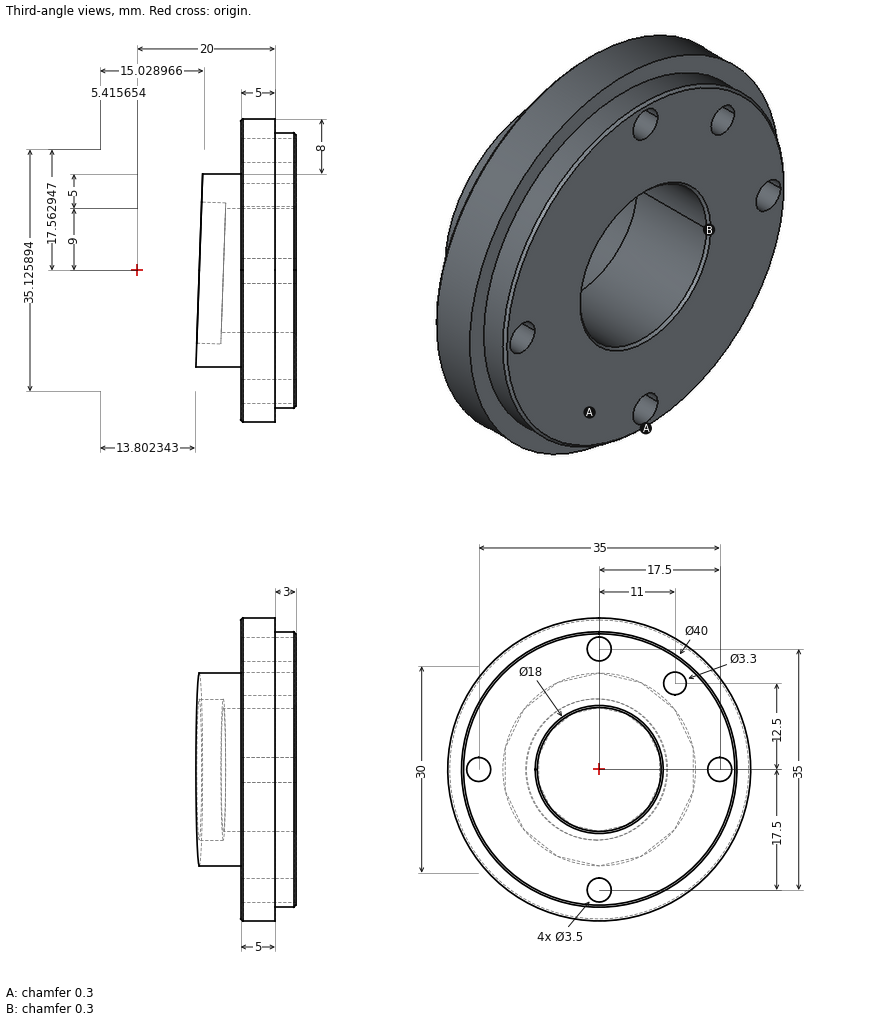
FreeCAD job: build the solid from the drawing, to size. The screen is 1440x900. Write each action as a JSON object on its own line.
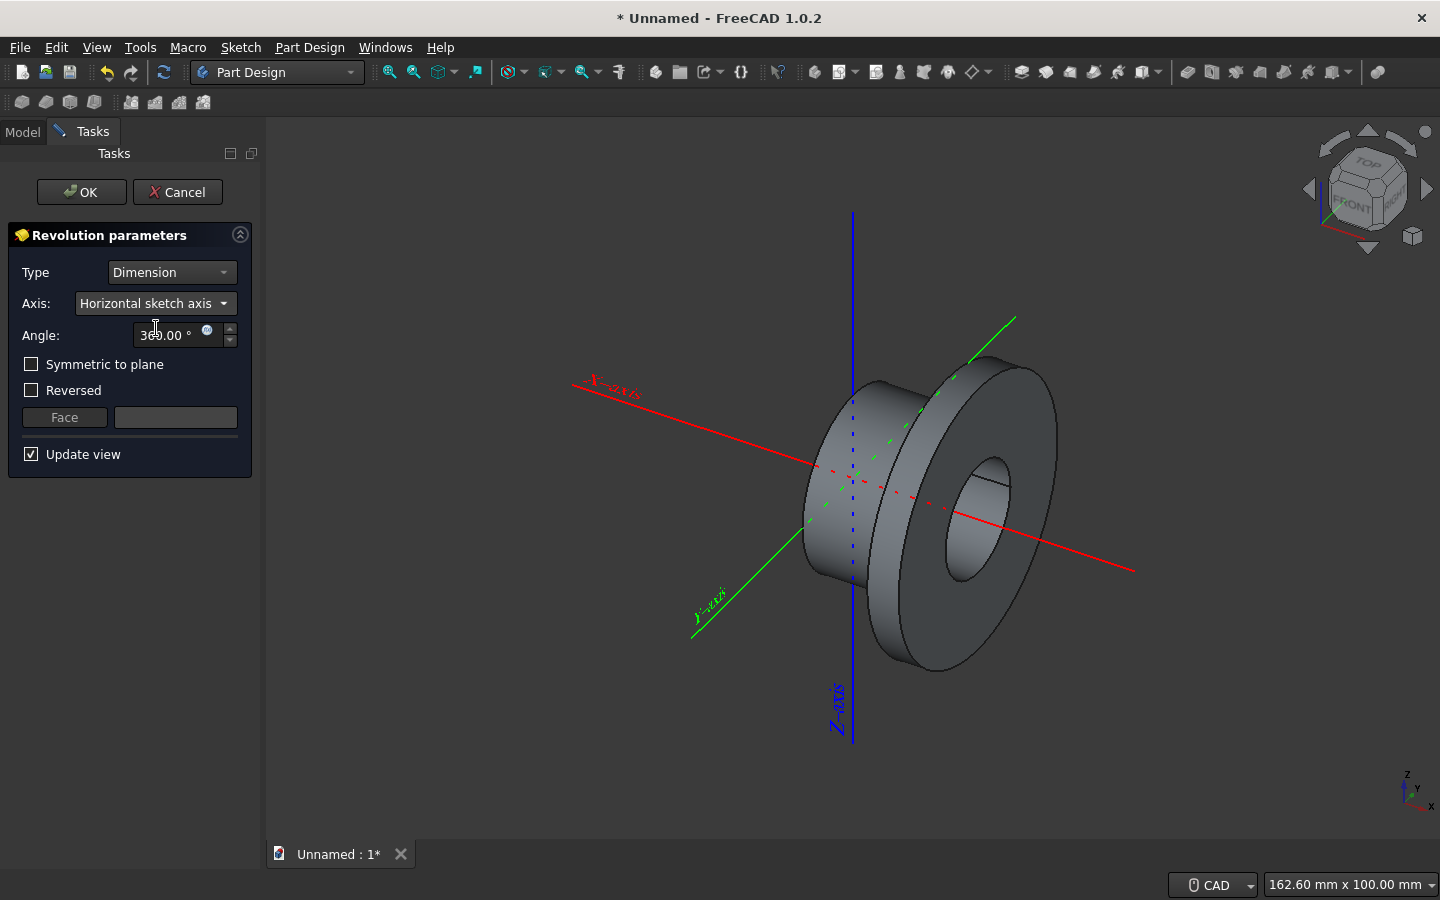
{"action": "left_click", "coordinate": [82, 192]}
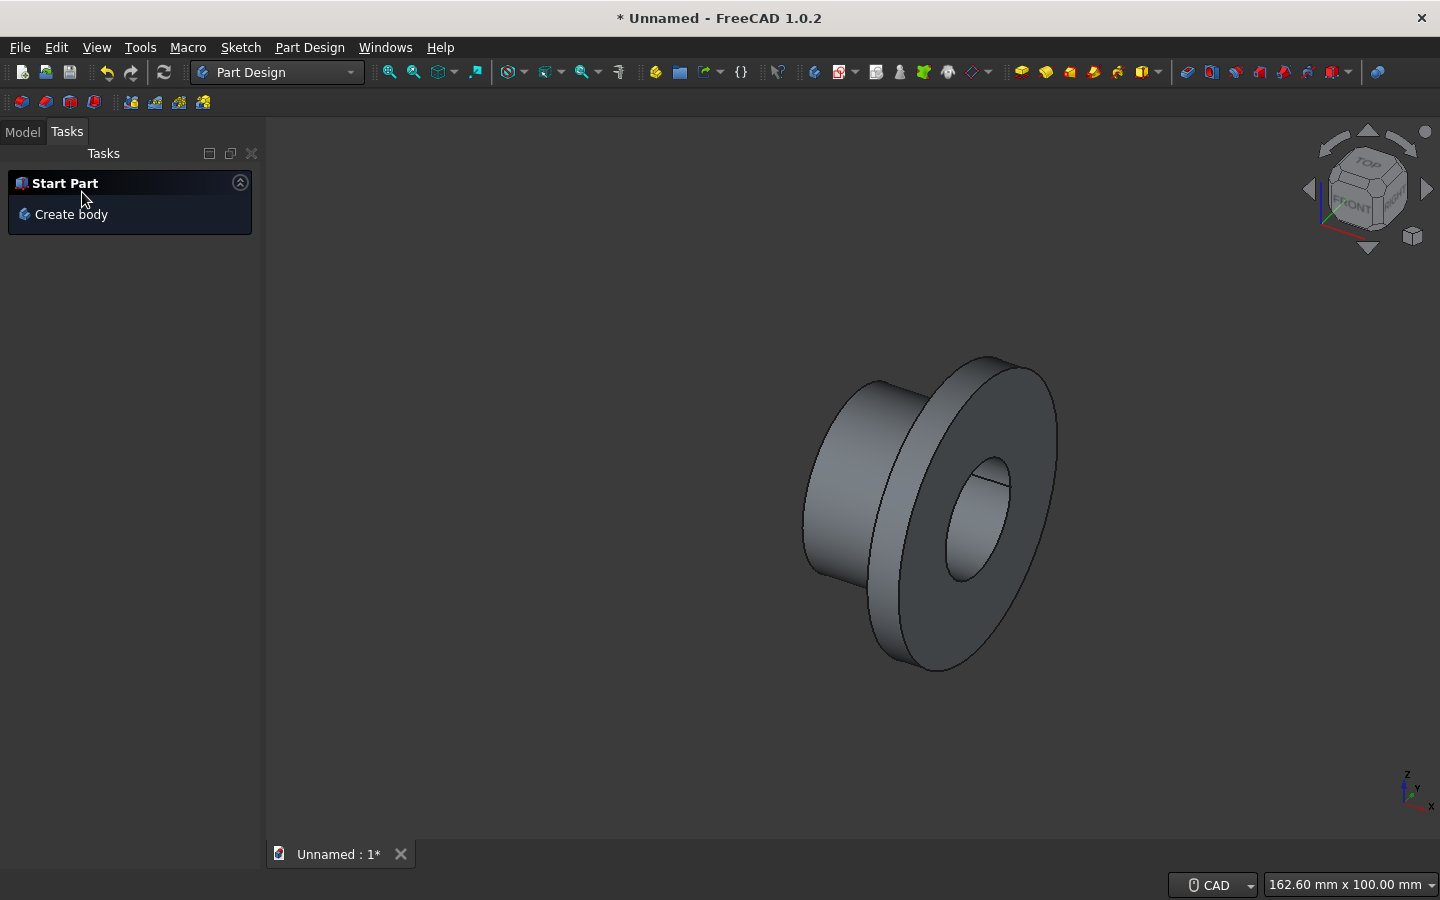
{"action": "left_click", "coordinate": [840, 72]}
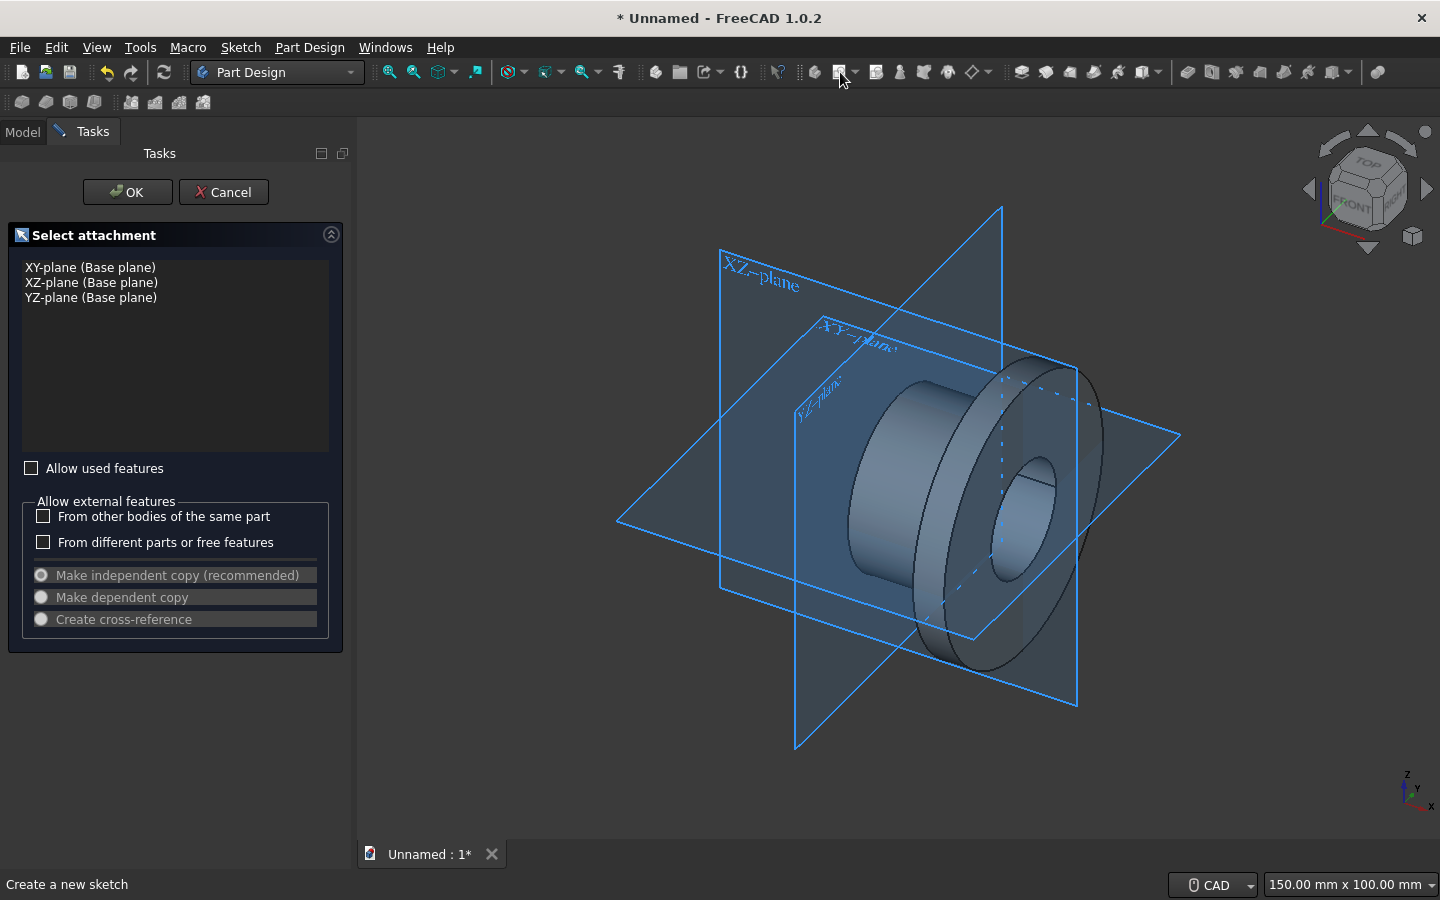
{"action": "left_click", "coordinate": [82, 268]}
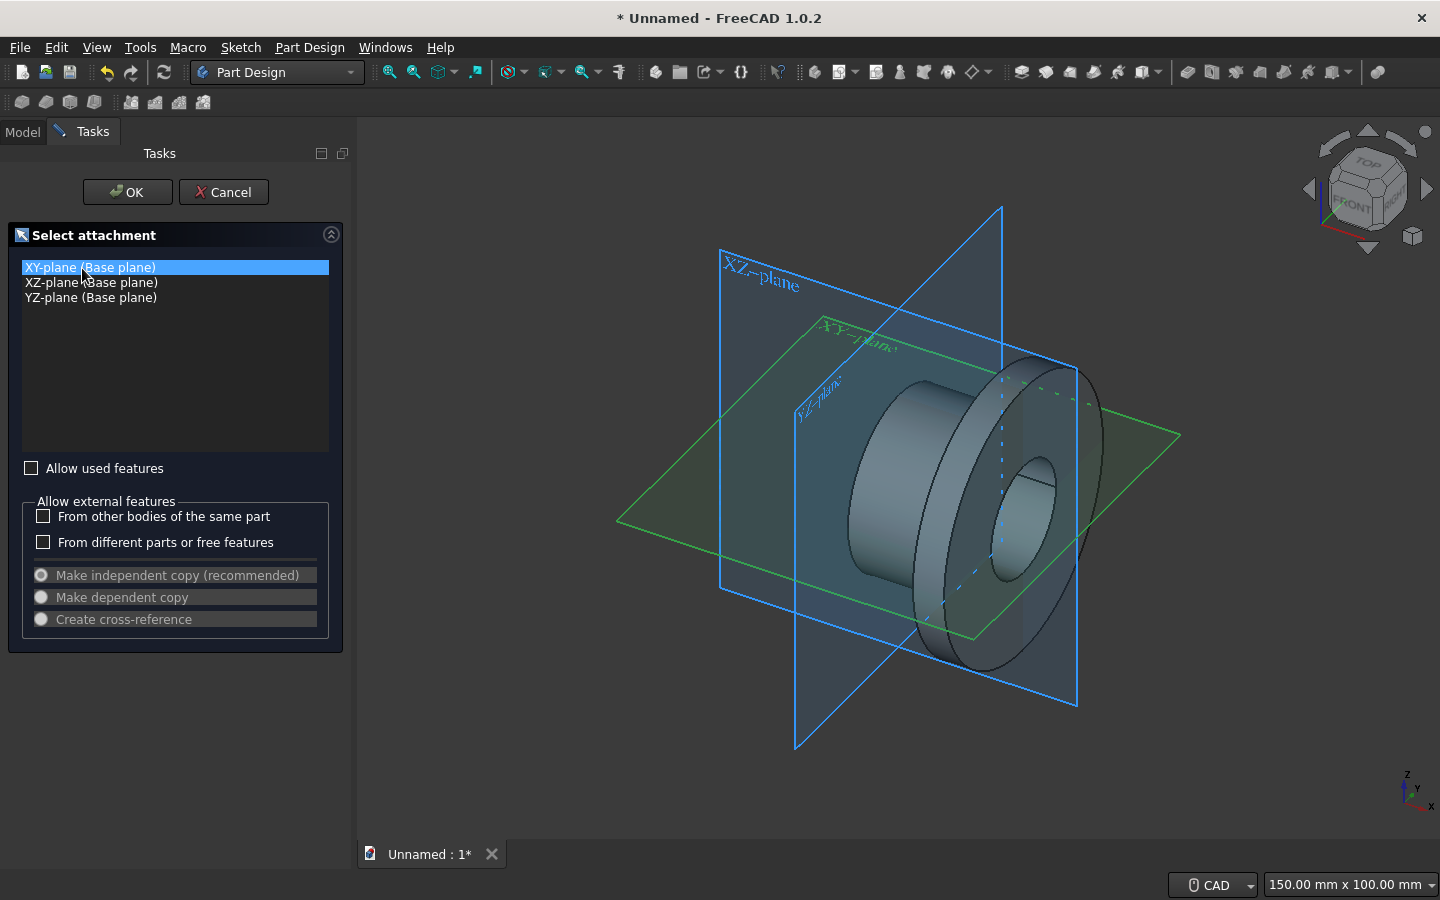
{"action": "left_click", "coordinate": [128, 192]}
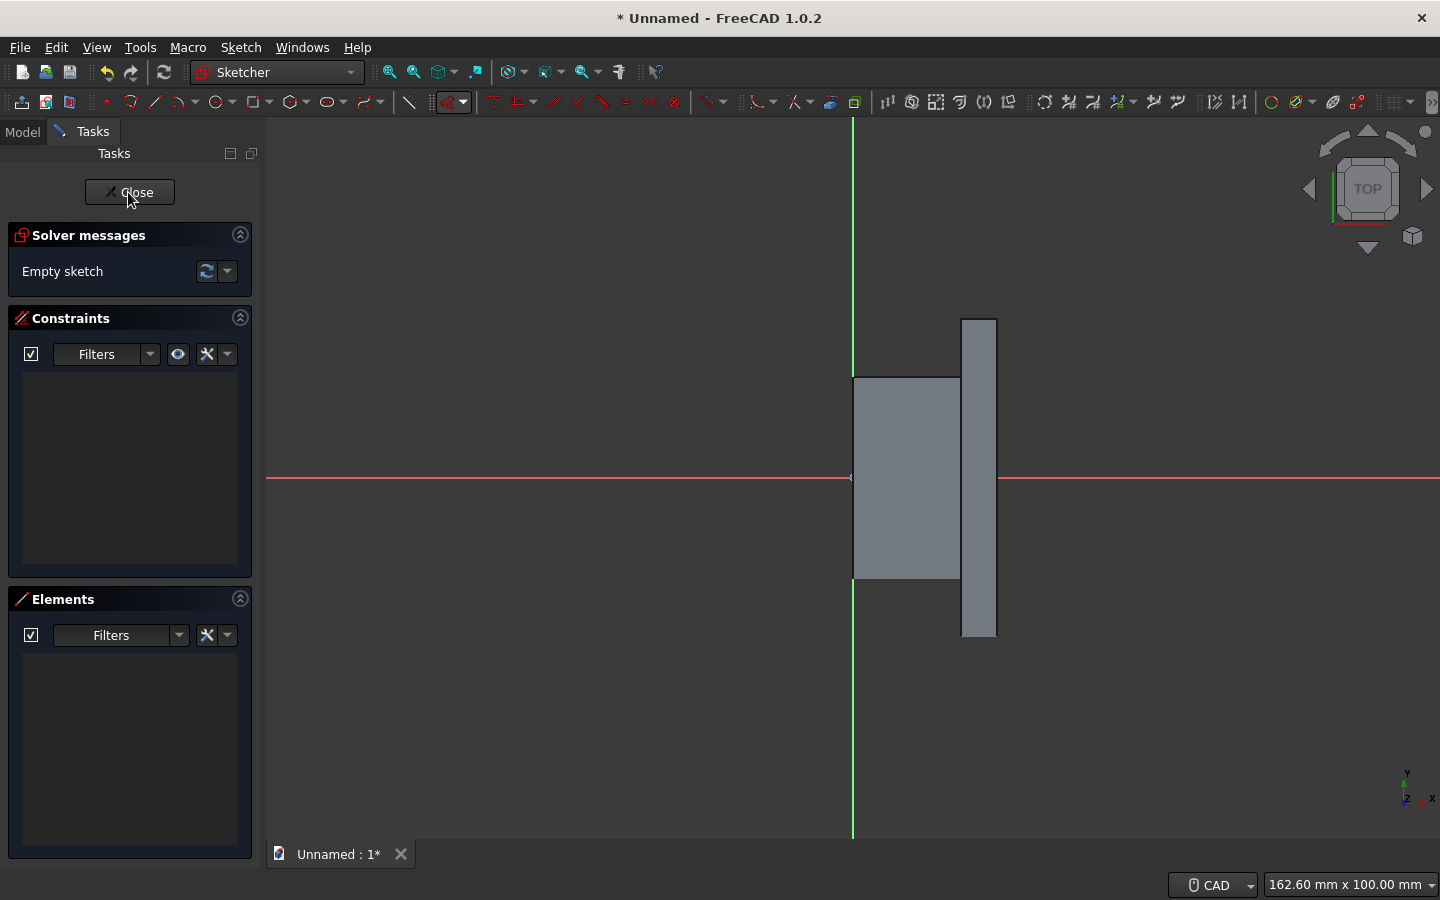
{"action": "key", "text": "q s"}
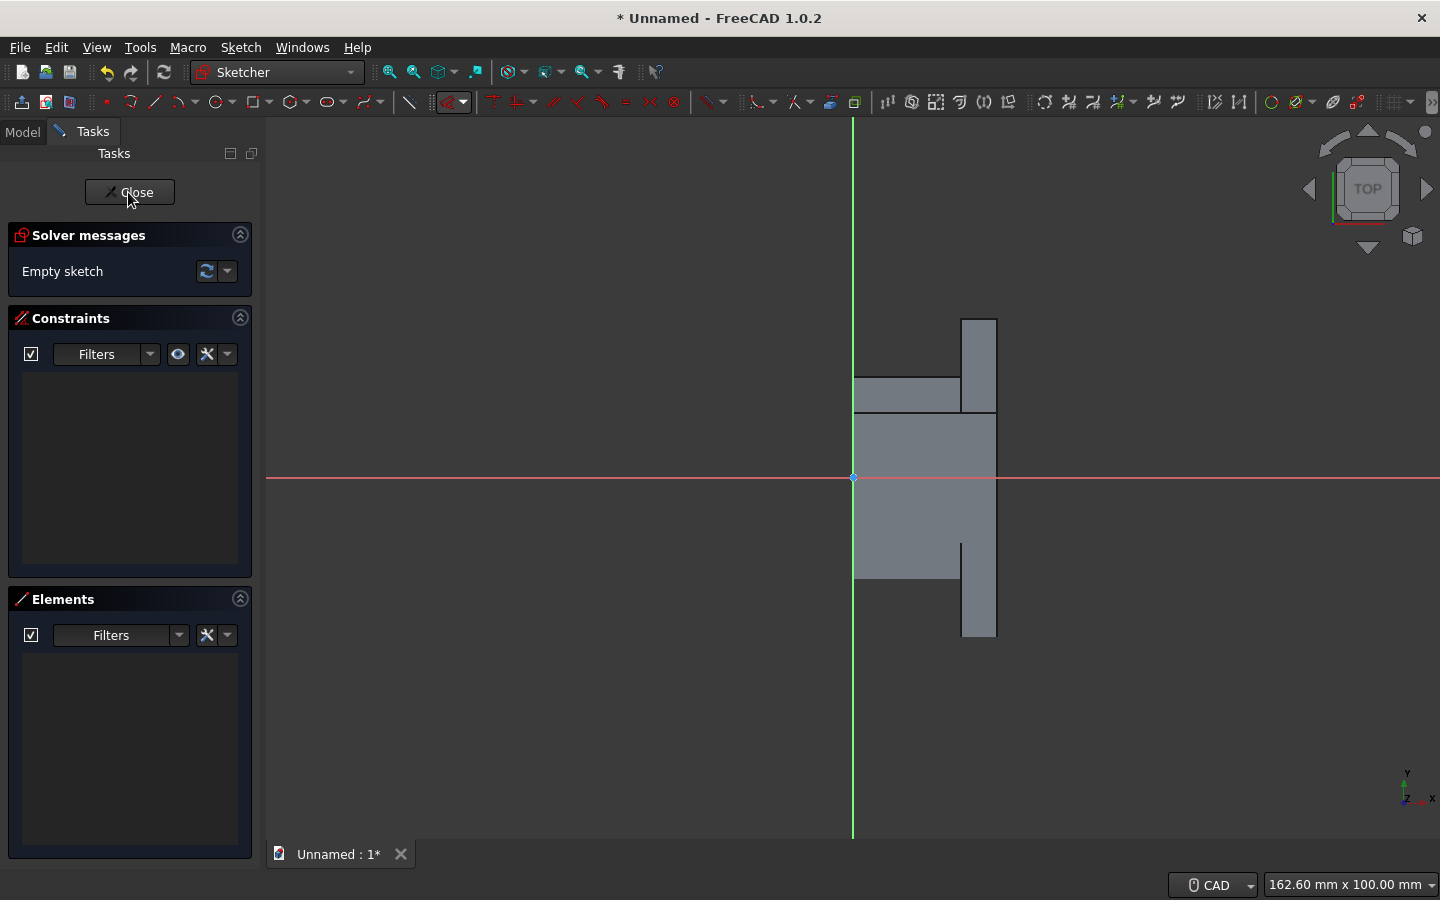
{"action": "scroll", "coordinate": [970, 478], "scroll_direction": "up", "scroll_amount": 3}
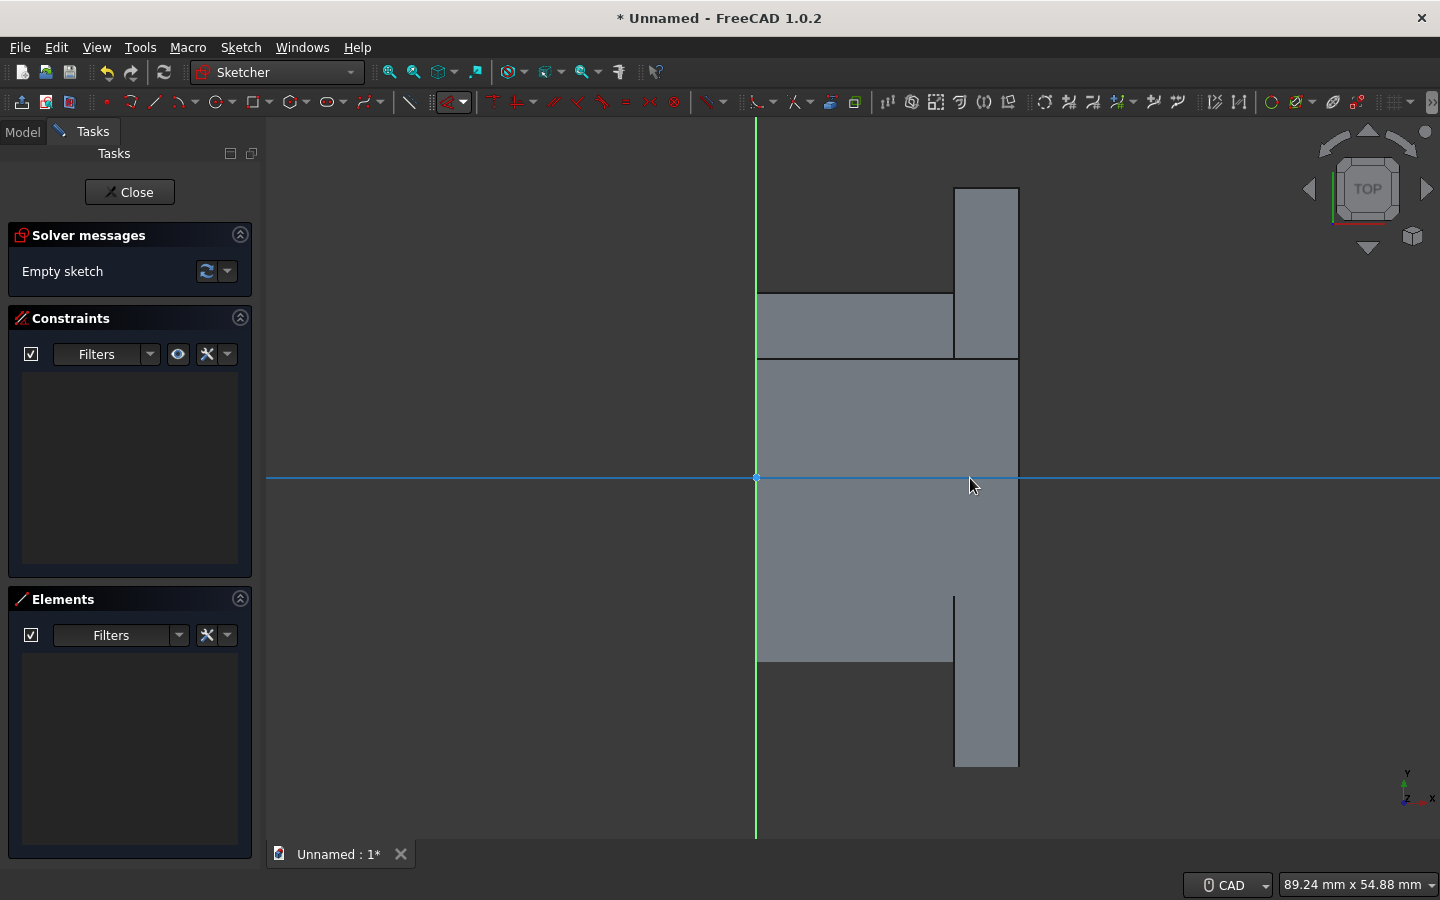
{"action": "left_click", "coordinate": [132, 102]}